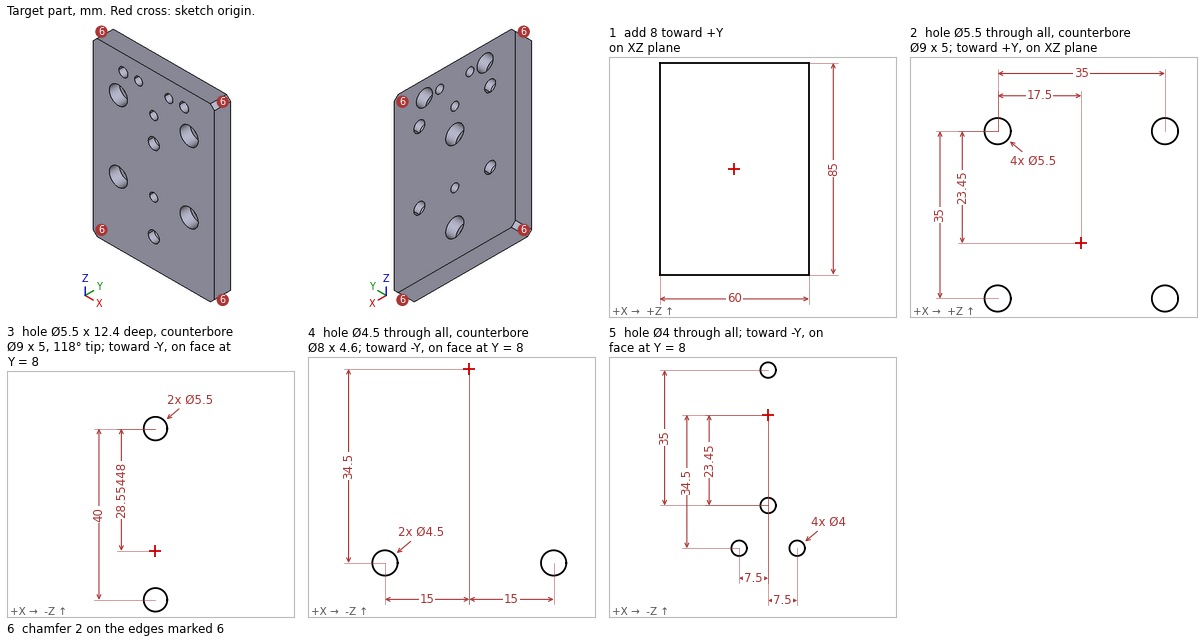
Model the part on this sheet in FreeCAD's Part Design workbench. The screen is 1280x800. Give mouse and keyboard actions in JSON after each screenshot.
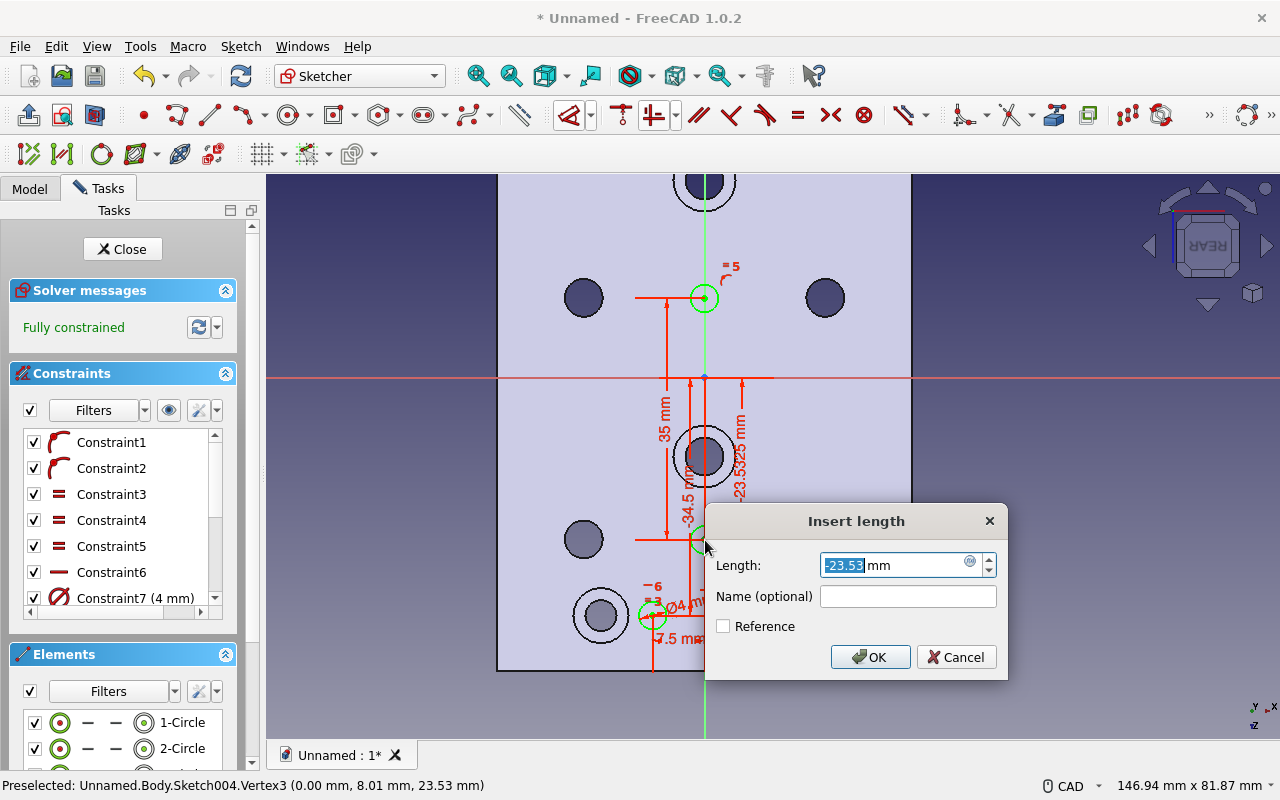
{"action": "type", "text": "-23.45"}
{"action": "key", "text": "Return"}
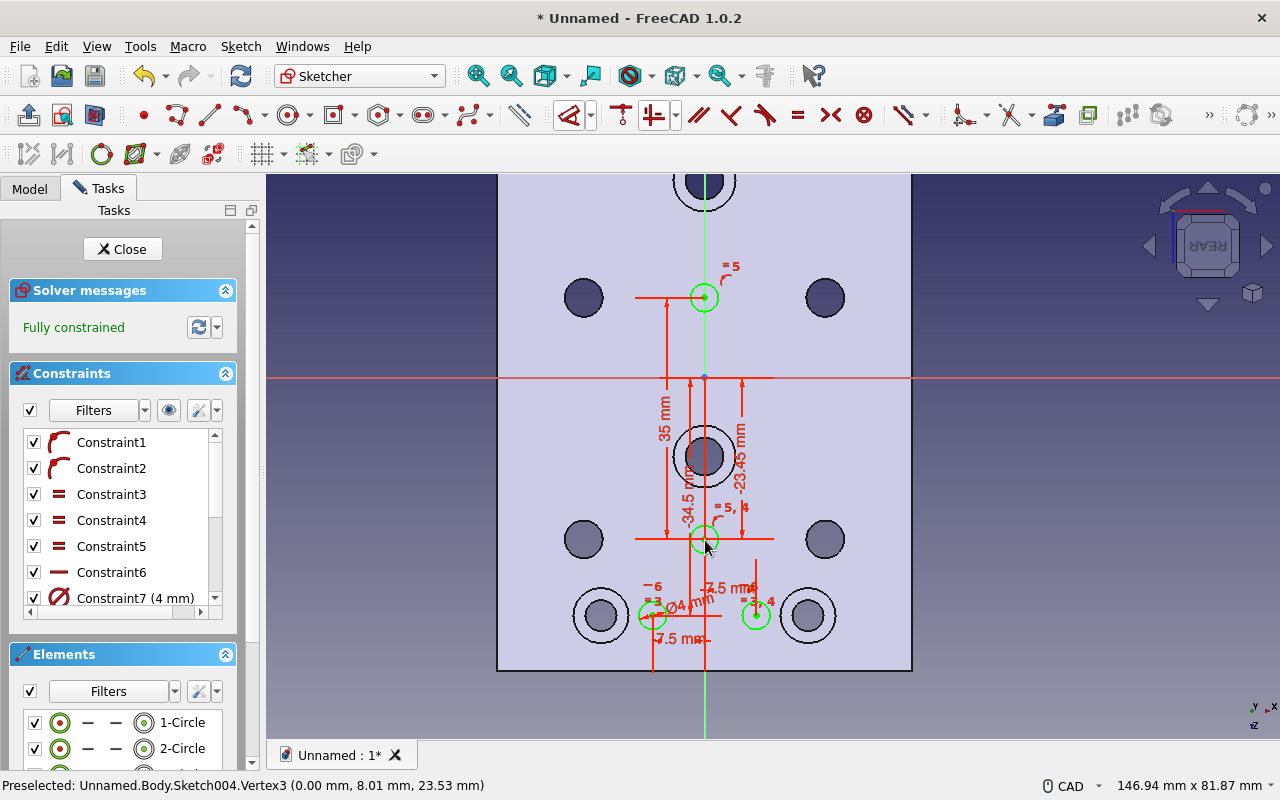
{"action": "left_click", "coordinate": [123, 249]}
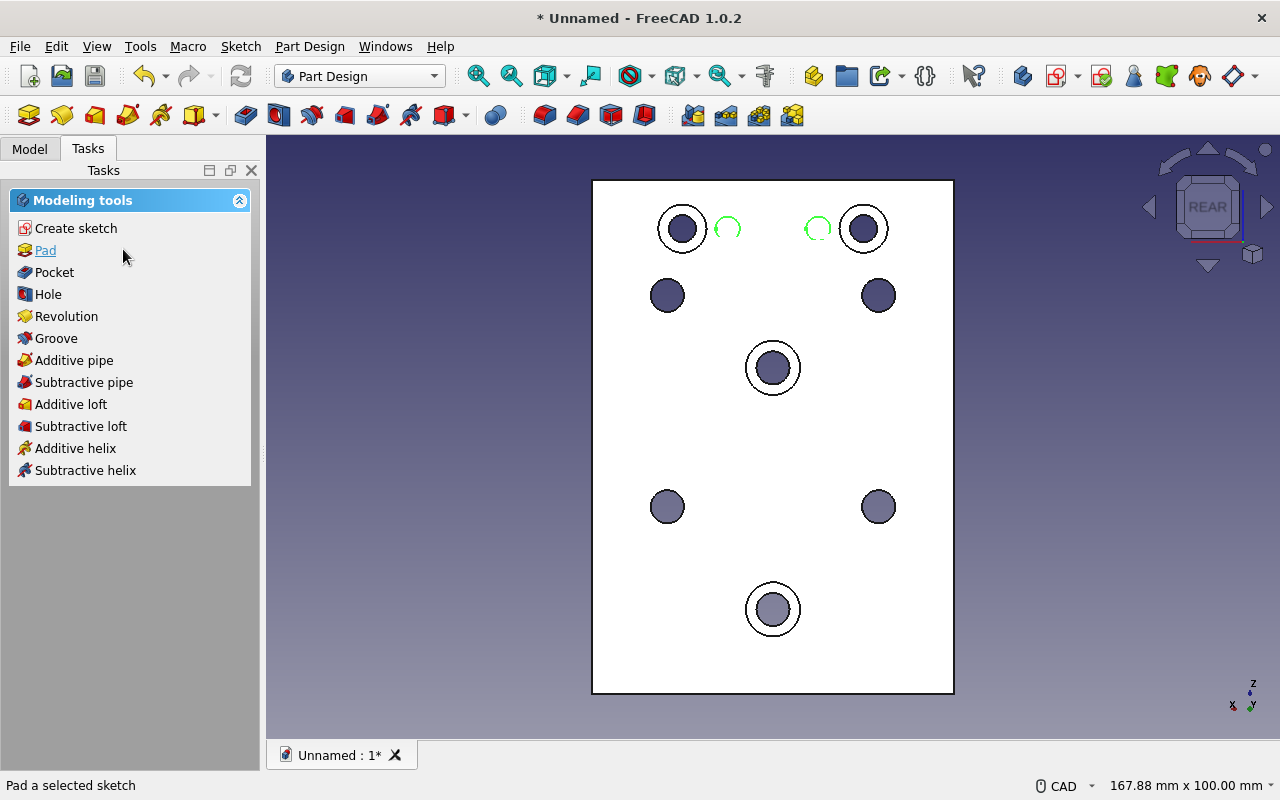
{"action": "left_click", "coordinate": [279, 116]}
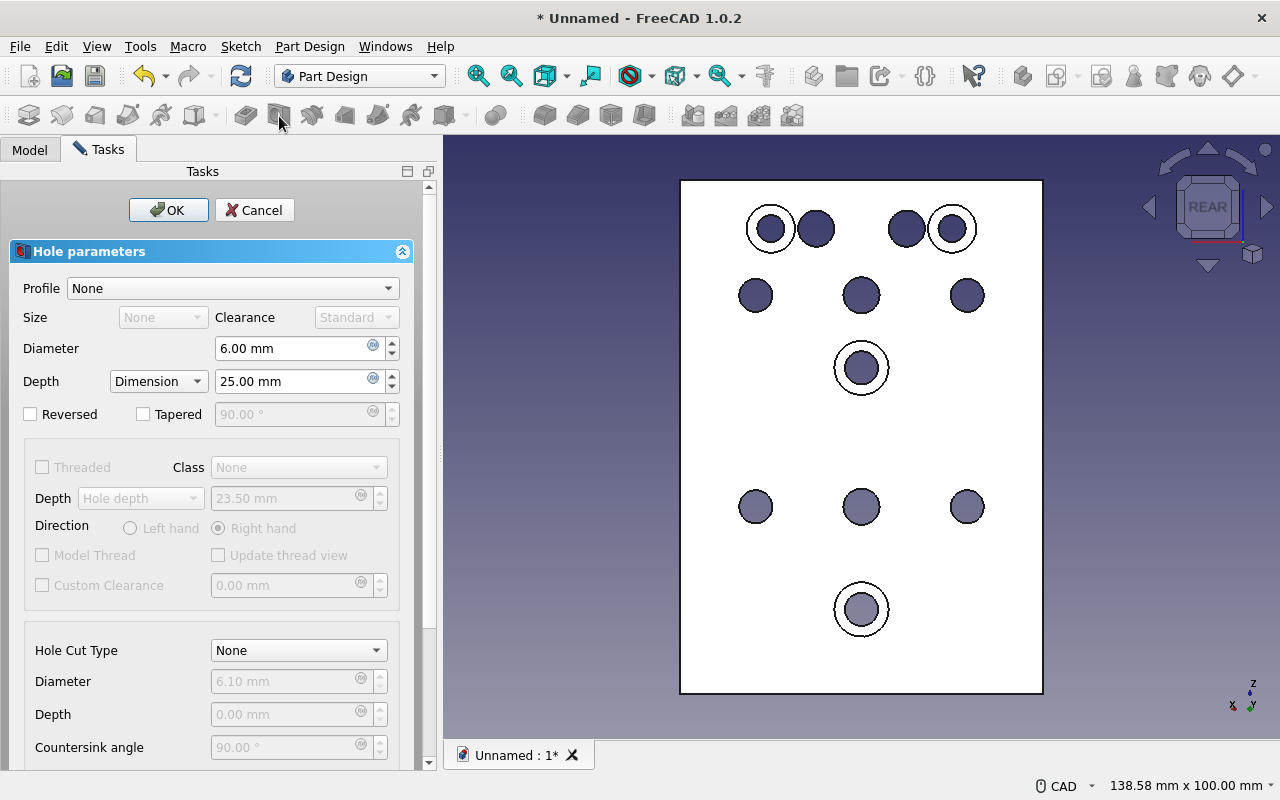
{"action": "triple_click", "coordinate": [300, 348]}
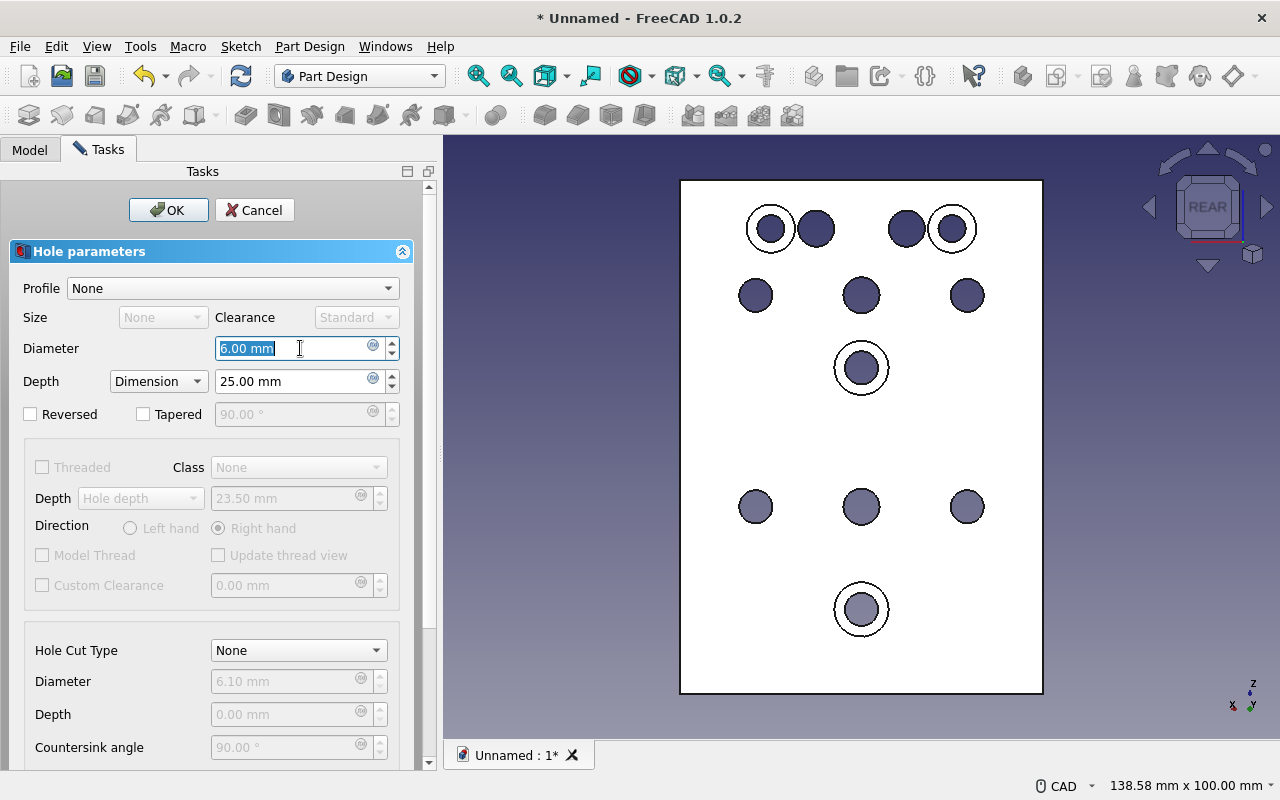
{"action": "type", "text": "4"}
{"action": "key", "text": "Tab"}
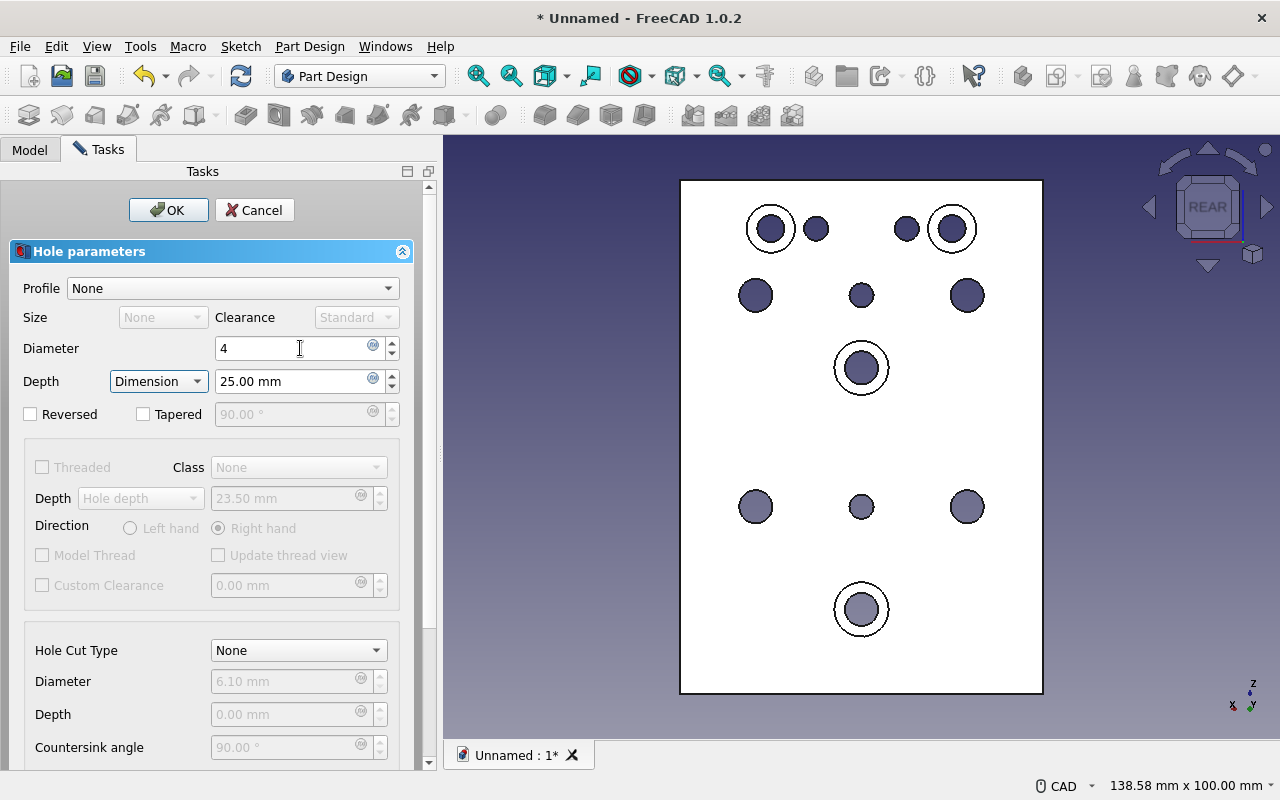
{"action": "left_click", "coordinate": [160, 382]}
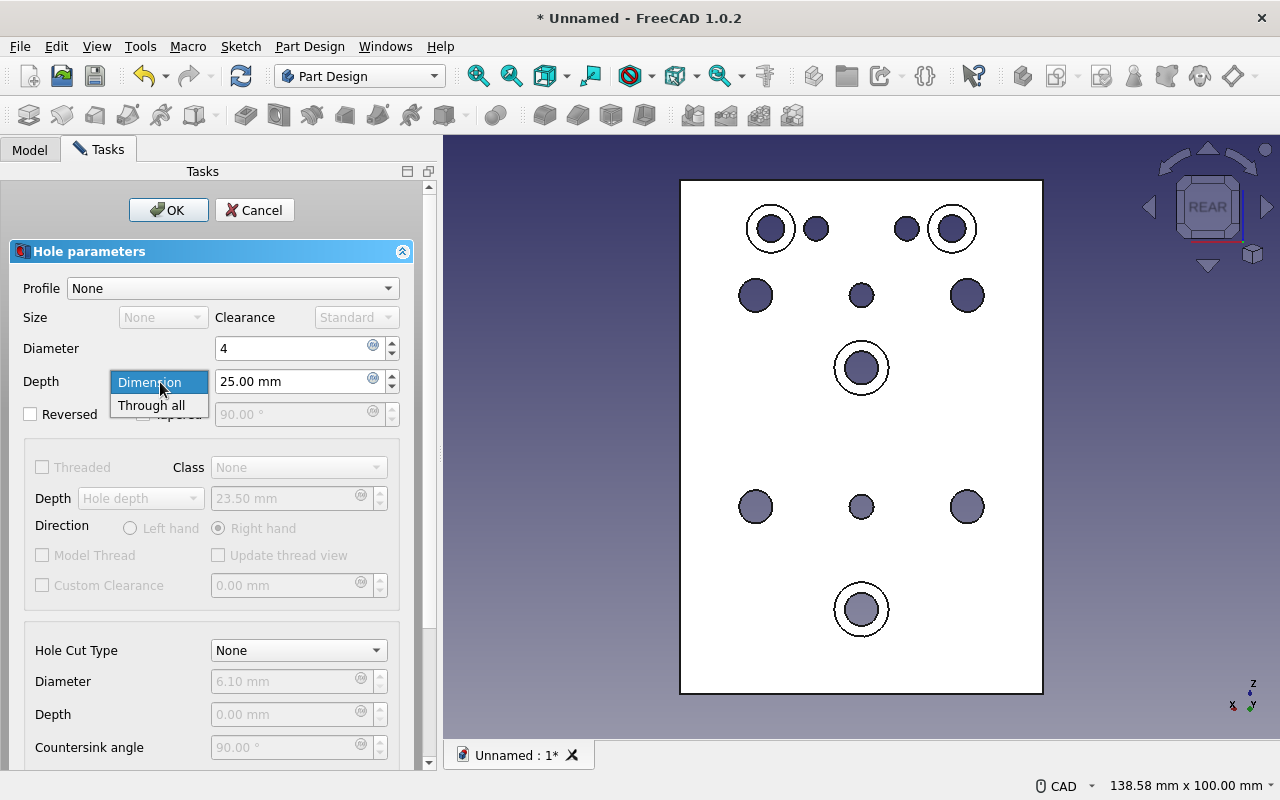
{"action": "left_click", "coordinate": [158, 406]}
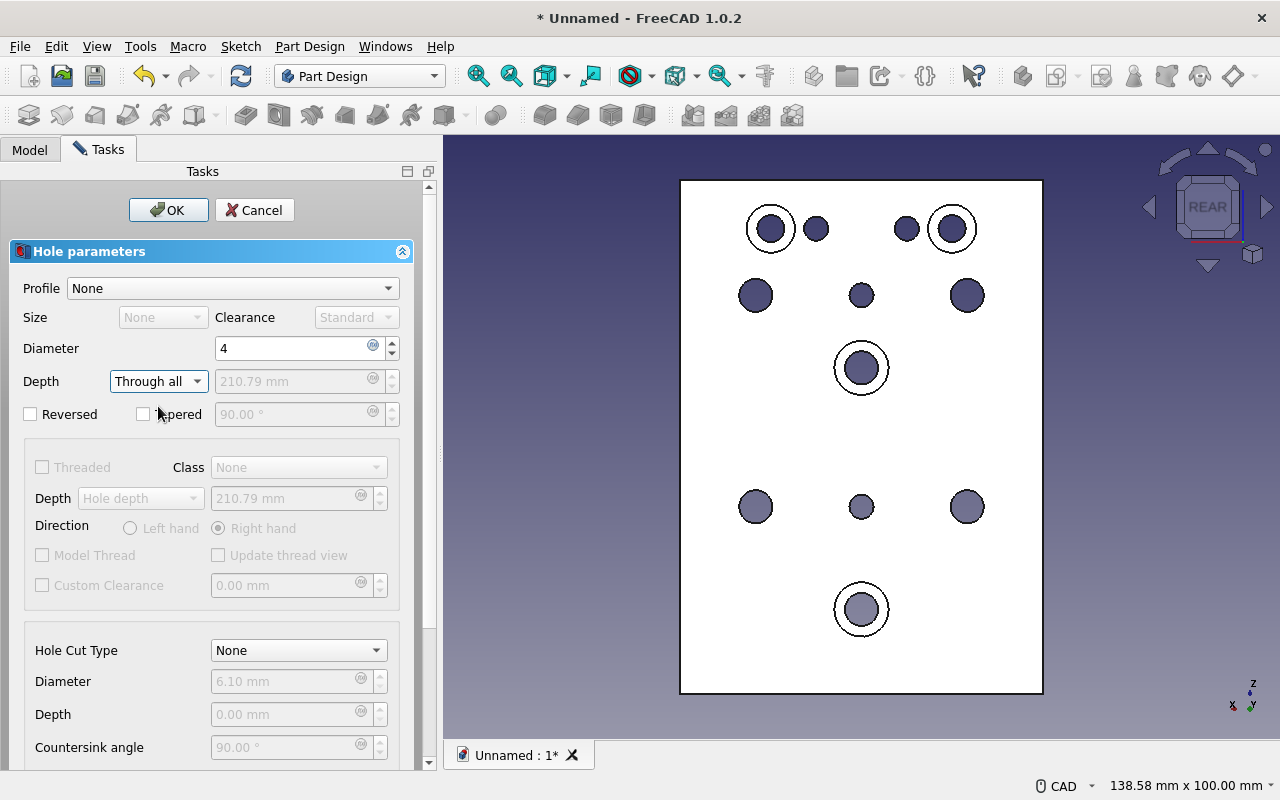
{"action": "left_click", "coordinate": [169, 210]}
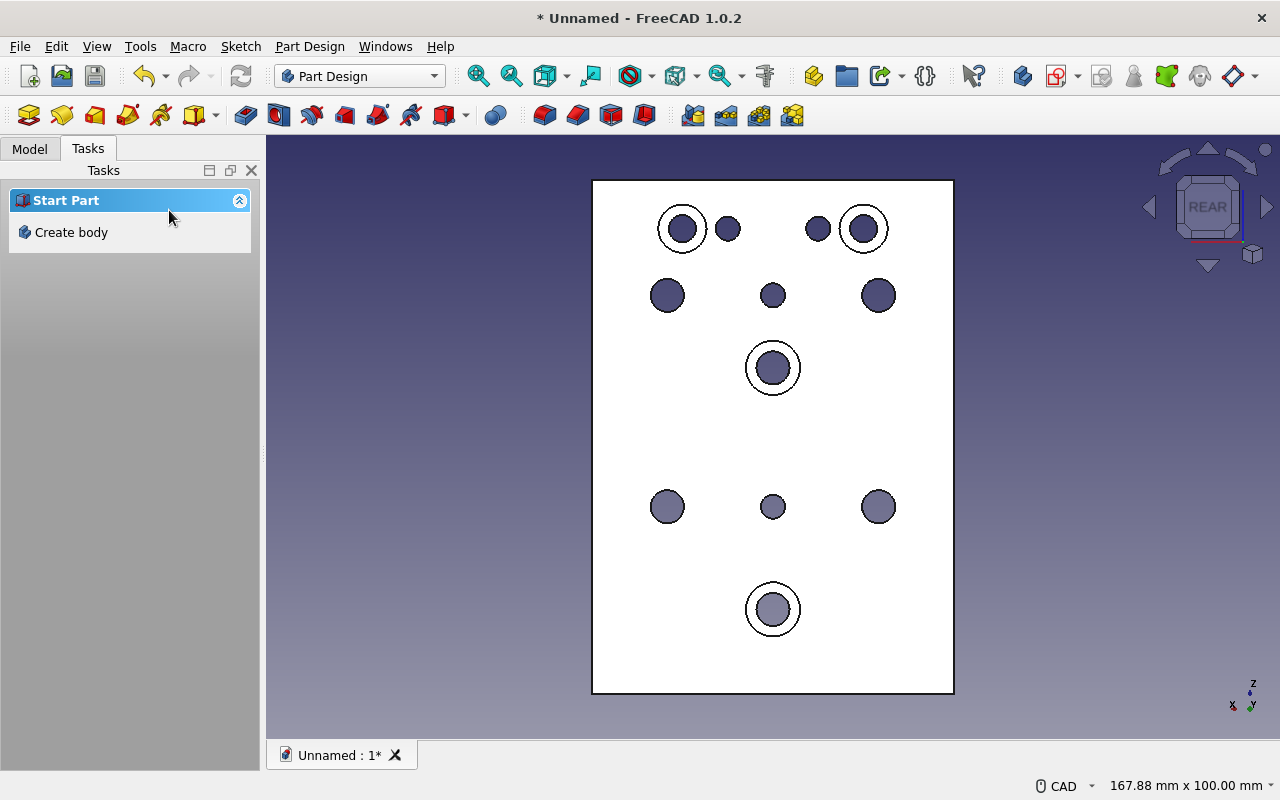
{"action": "key", "text": "0"}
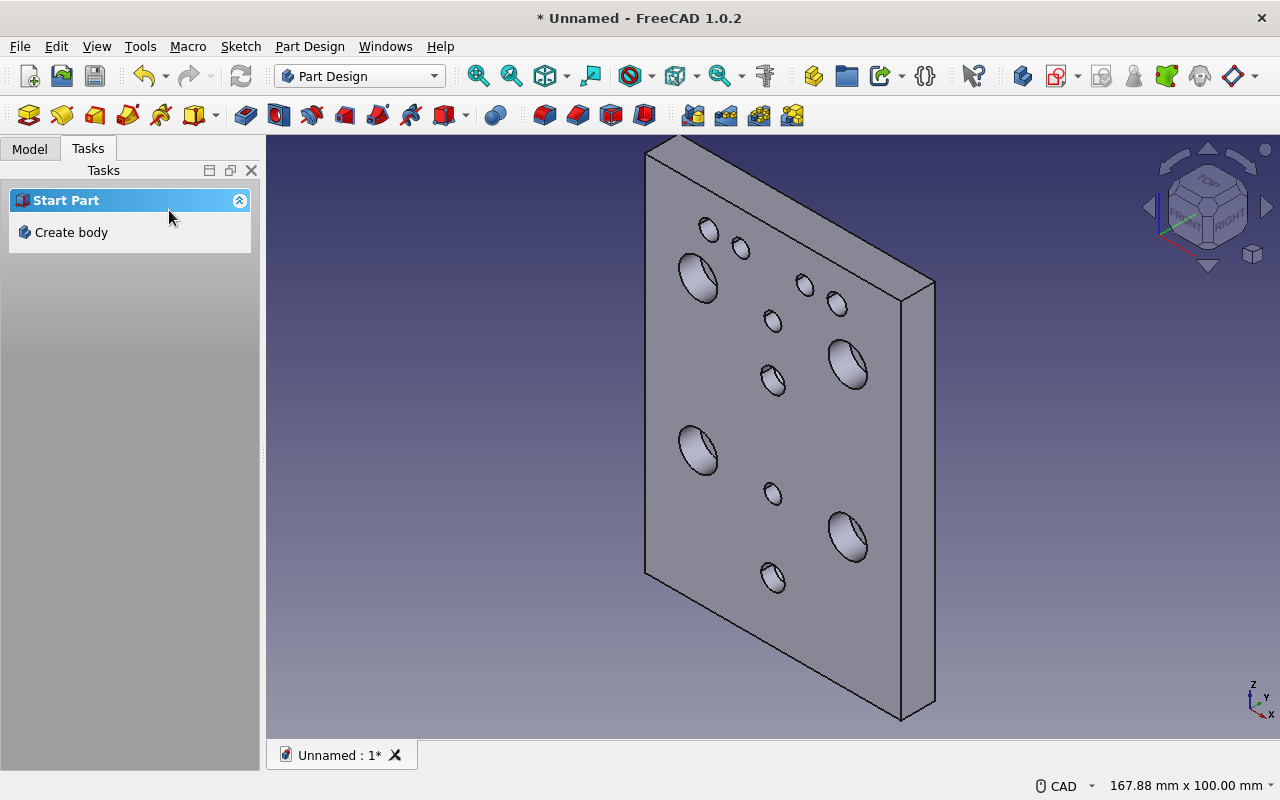
{"action": "left_click", "coordinate": [479, 76]}